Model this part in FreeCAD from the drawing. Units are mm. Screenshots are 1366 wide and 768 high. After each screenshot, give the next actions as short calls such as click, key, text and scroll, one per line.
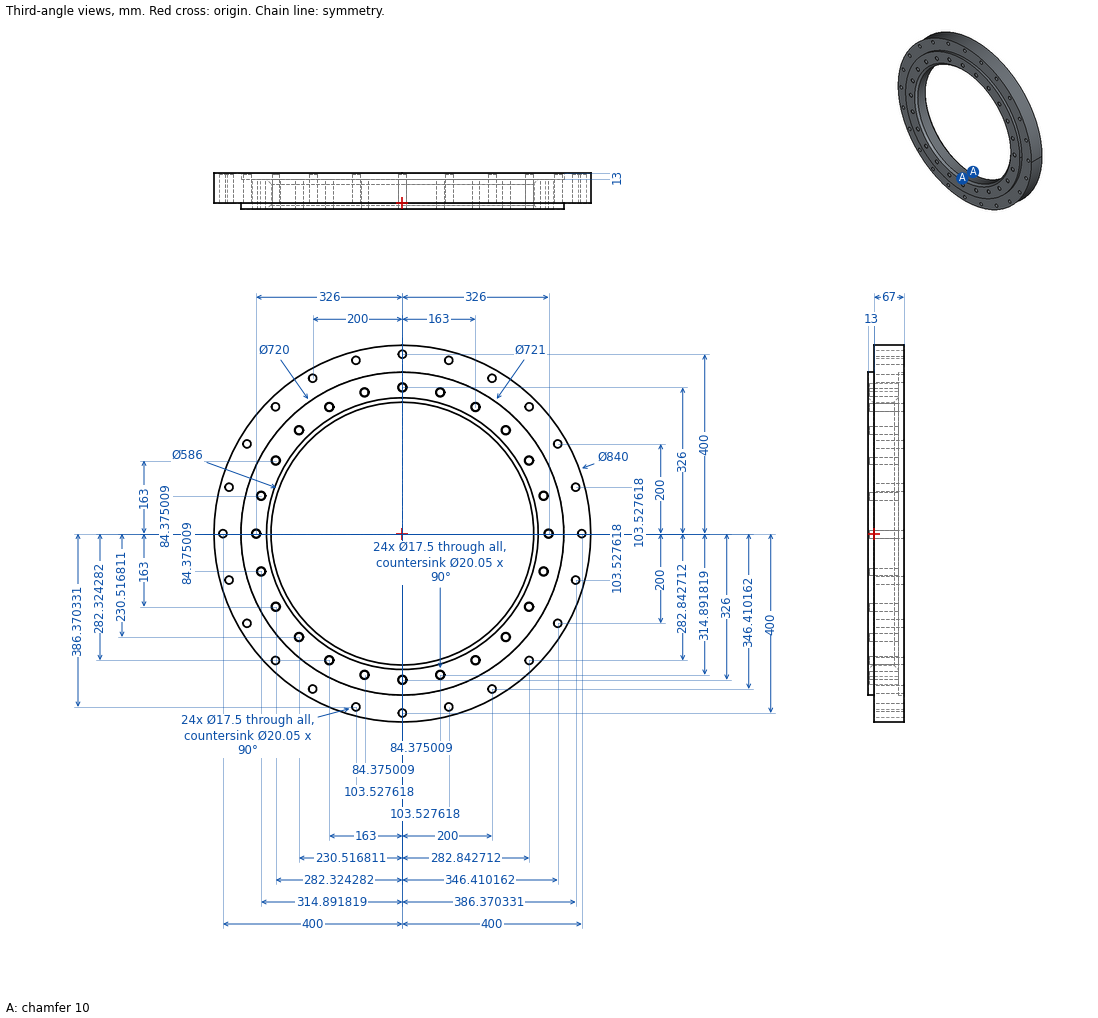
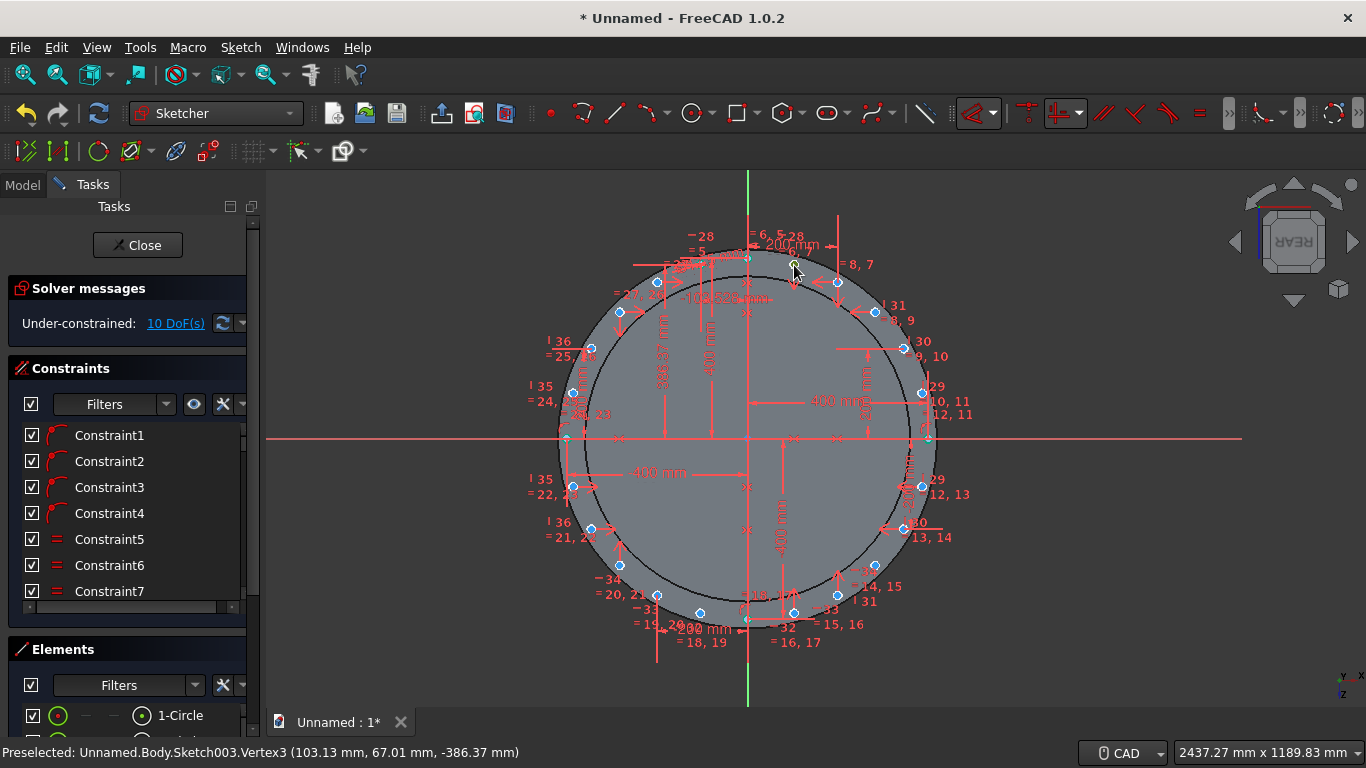
key(l)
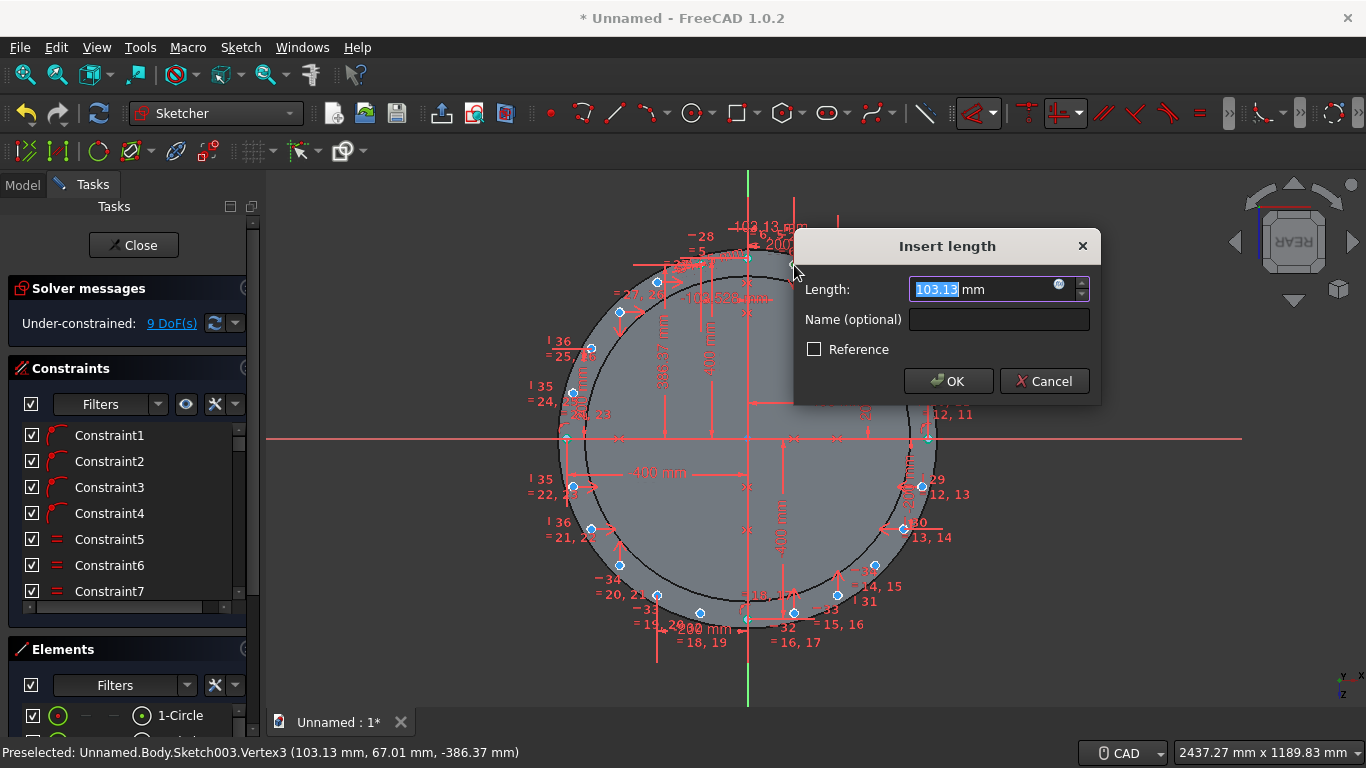
text(103.527618)
key(Return)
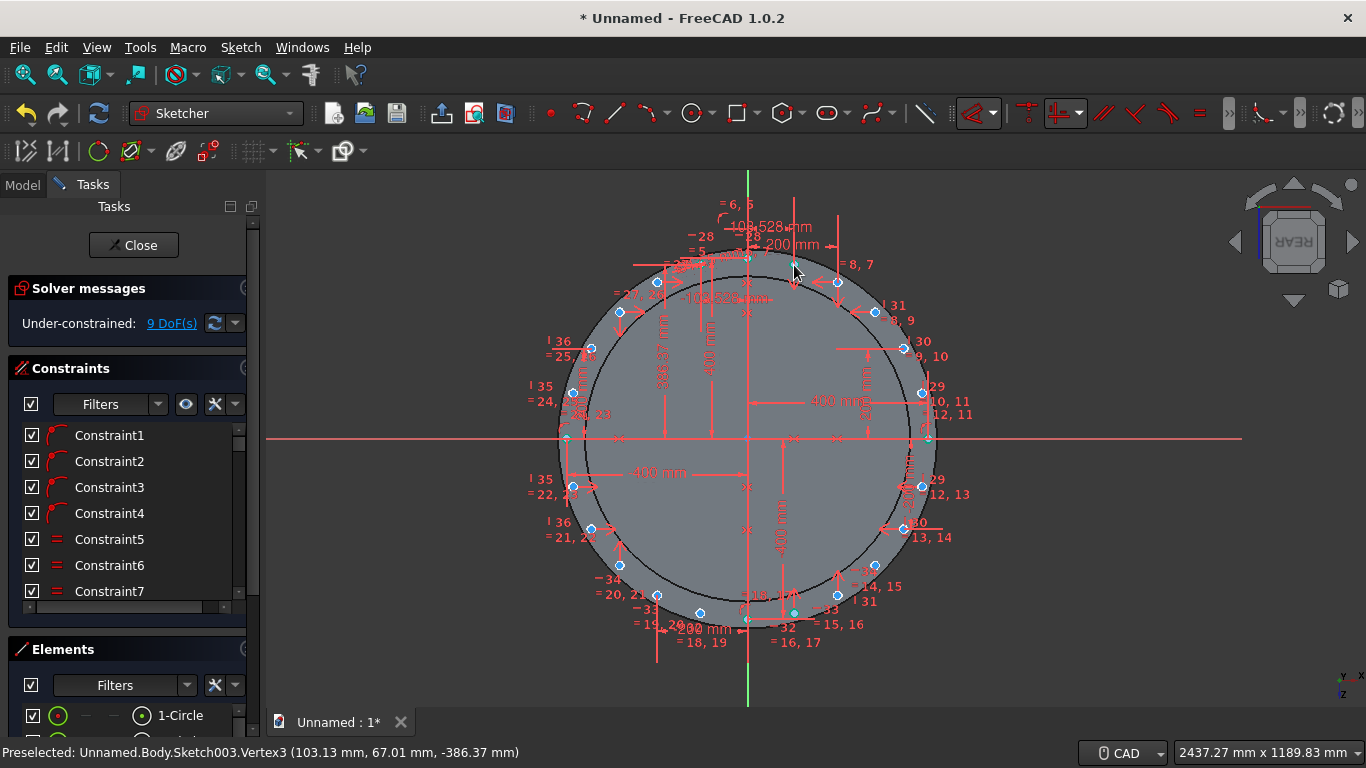
click(838, 282)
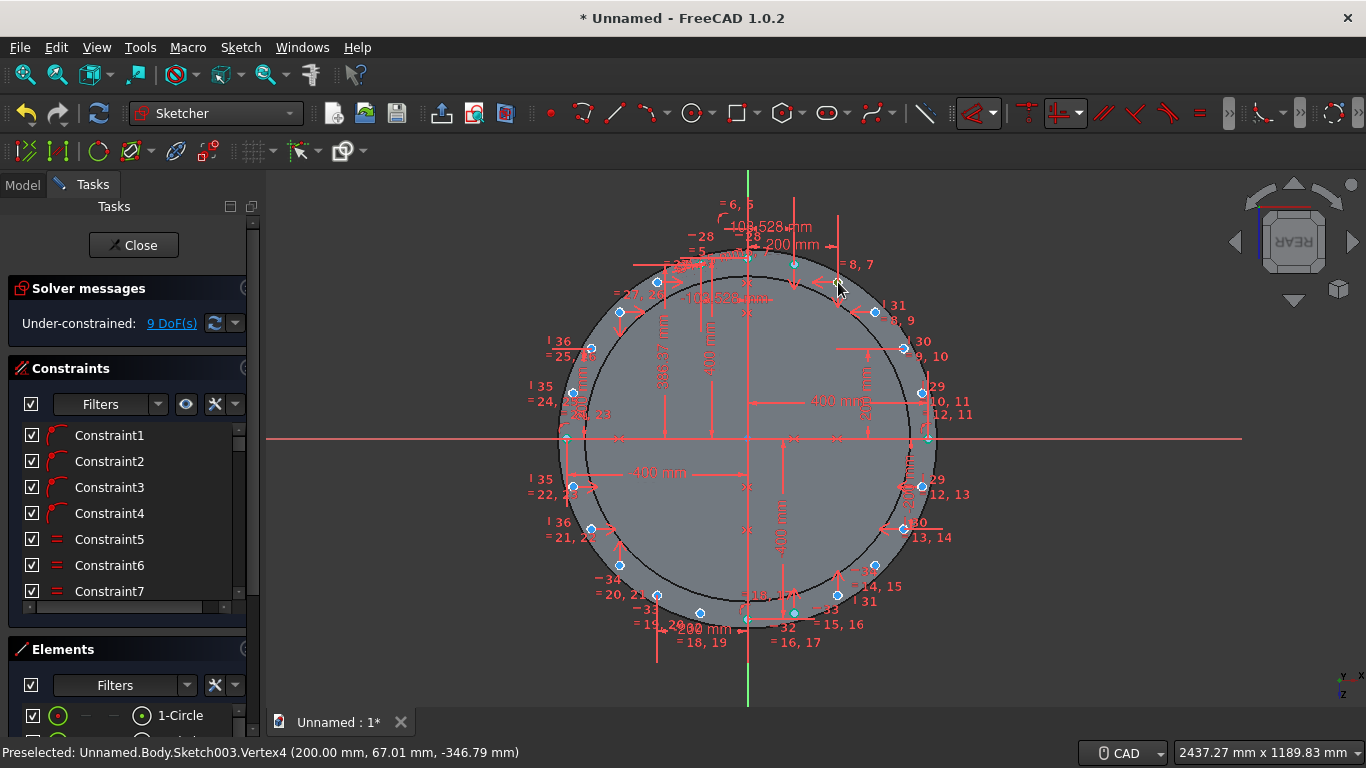
click(996, 114)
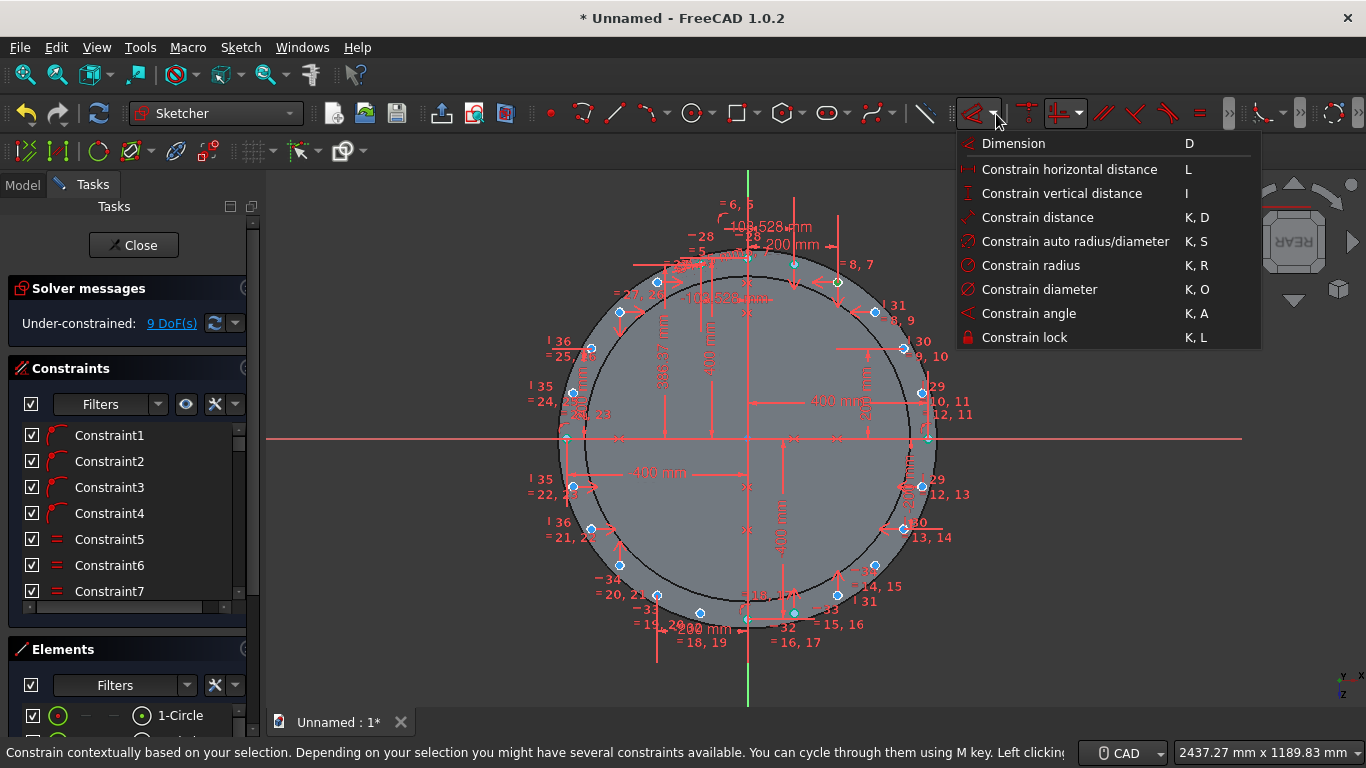
click(1109, 193)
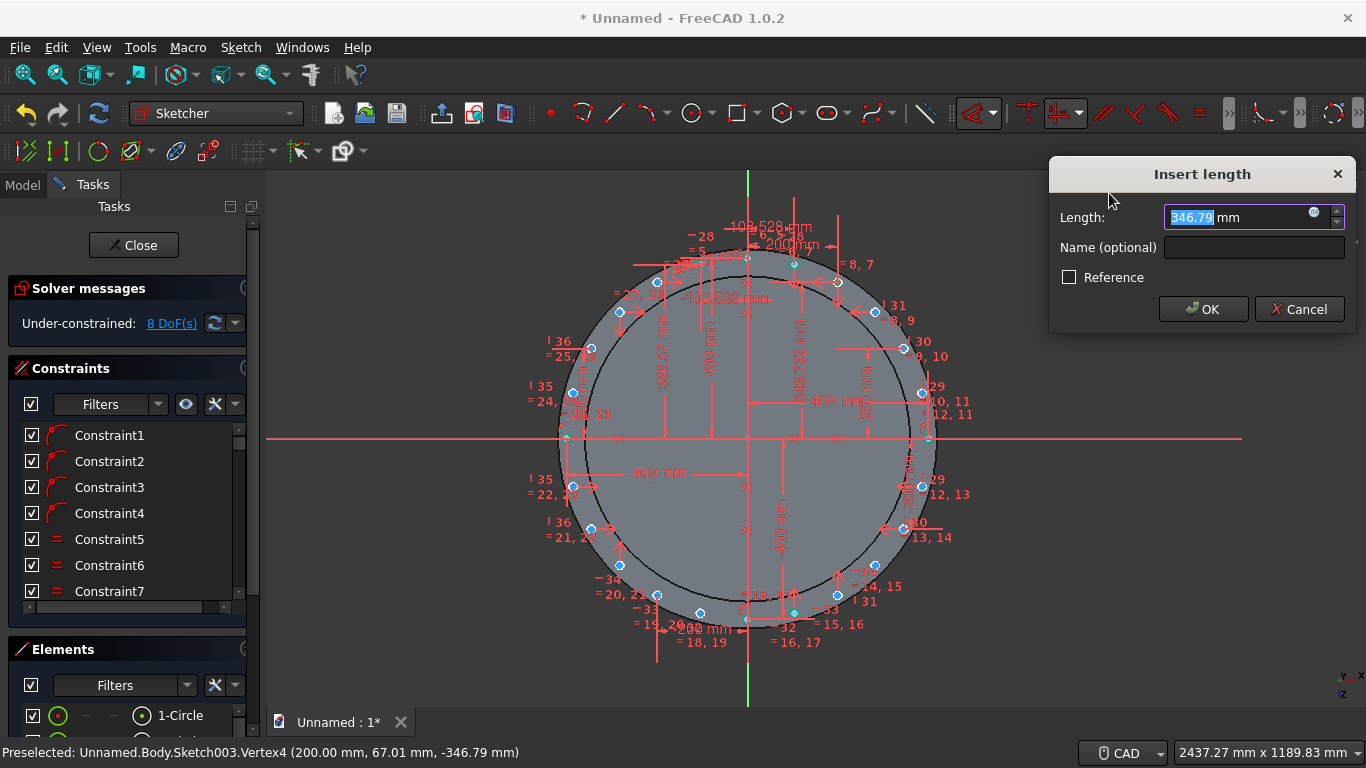
text(346.410162)
key(Return)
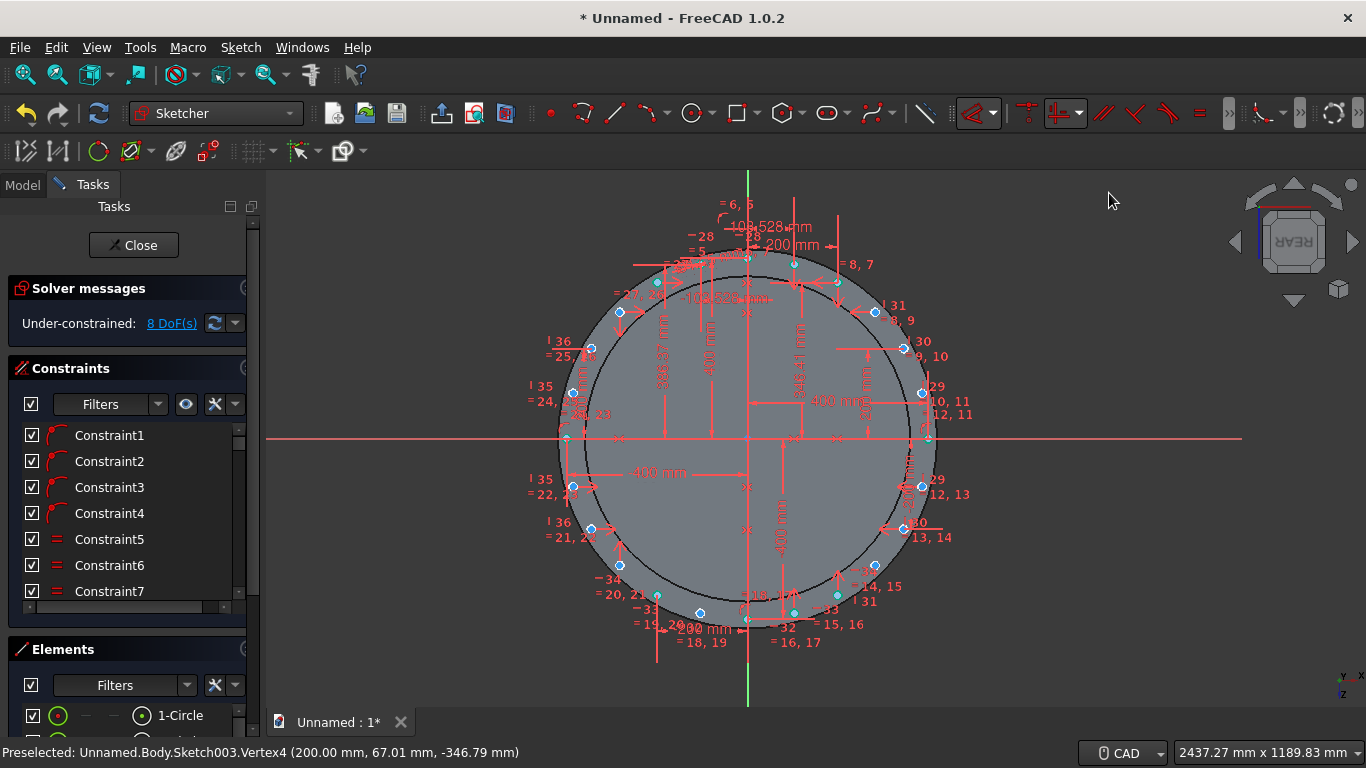
click(875, 312)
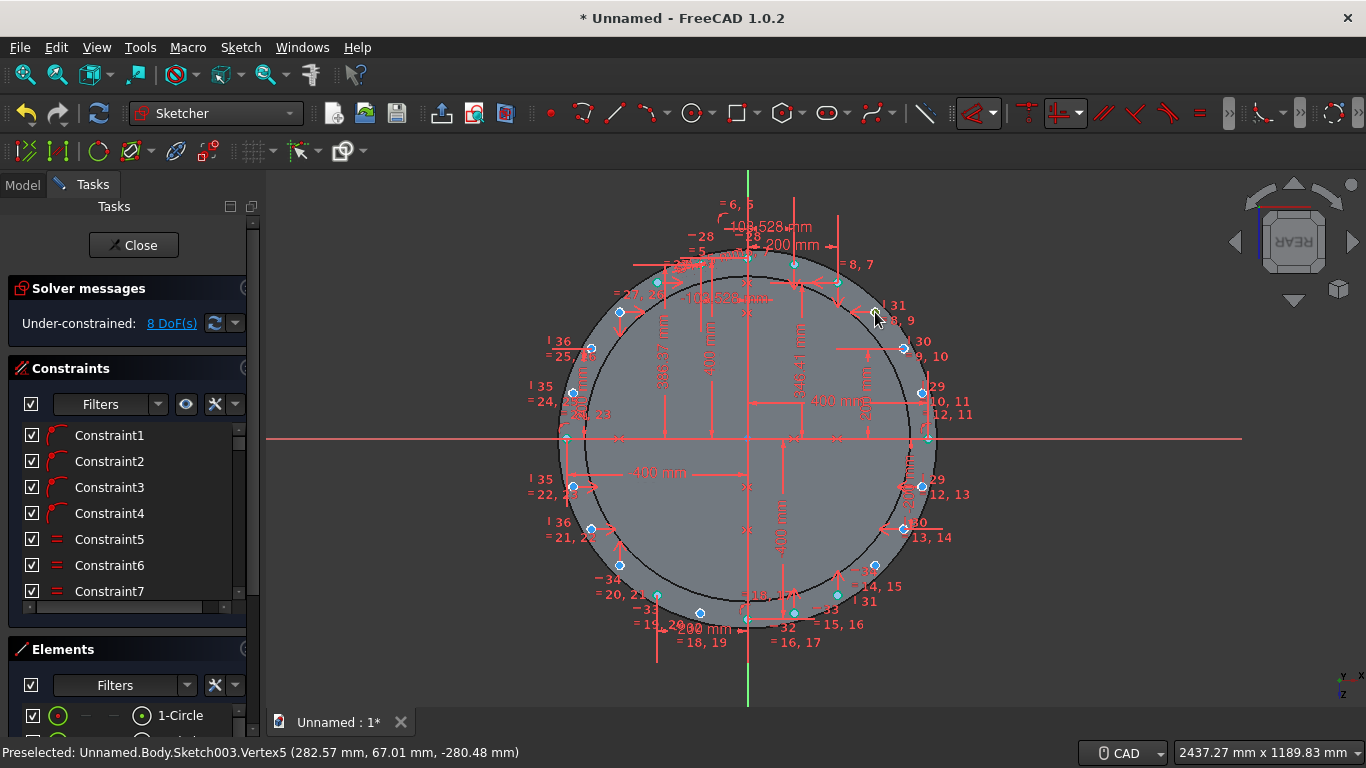
key(l)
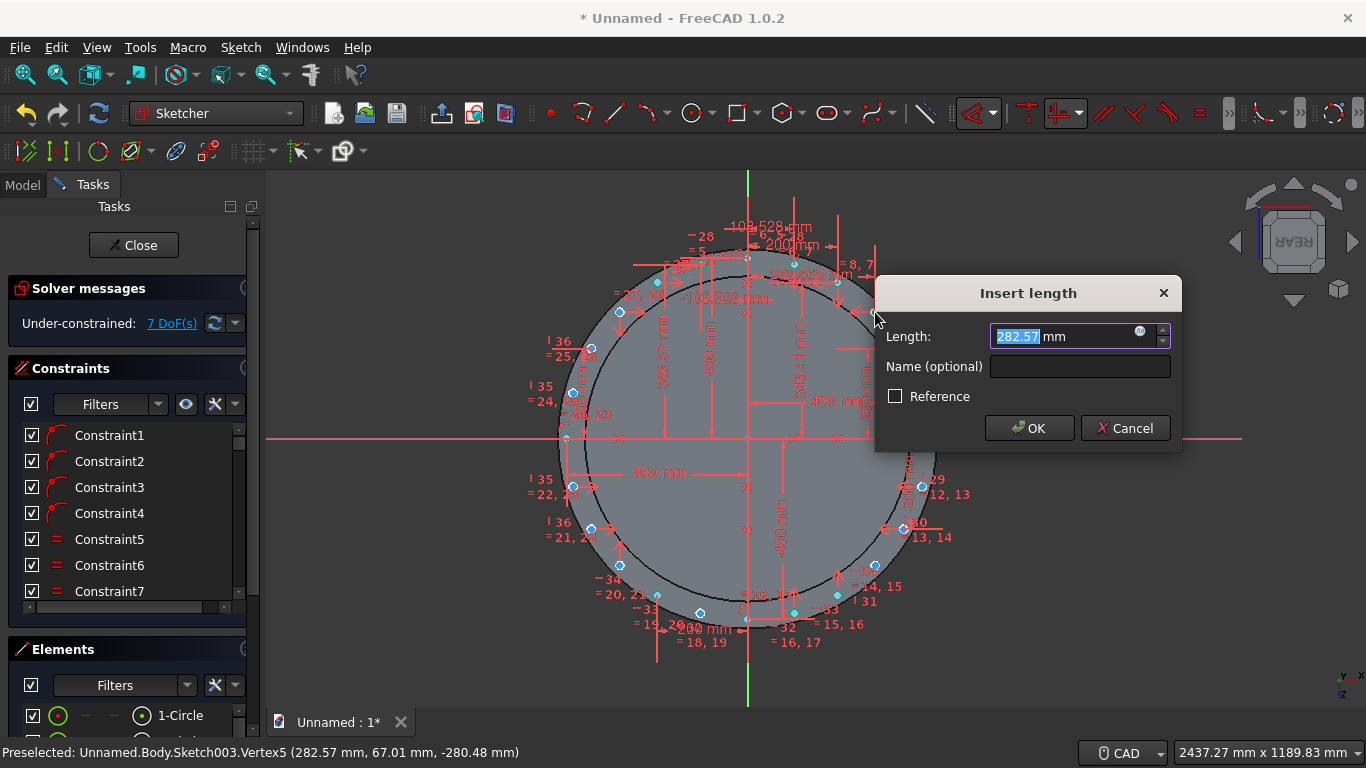
text(282.842712)
key(Return)